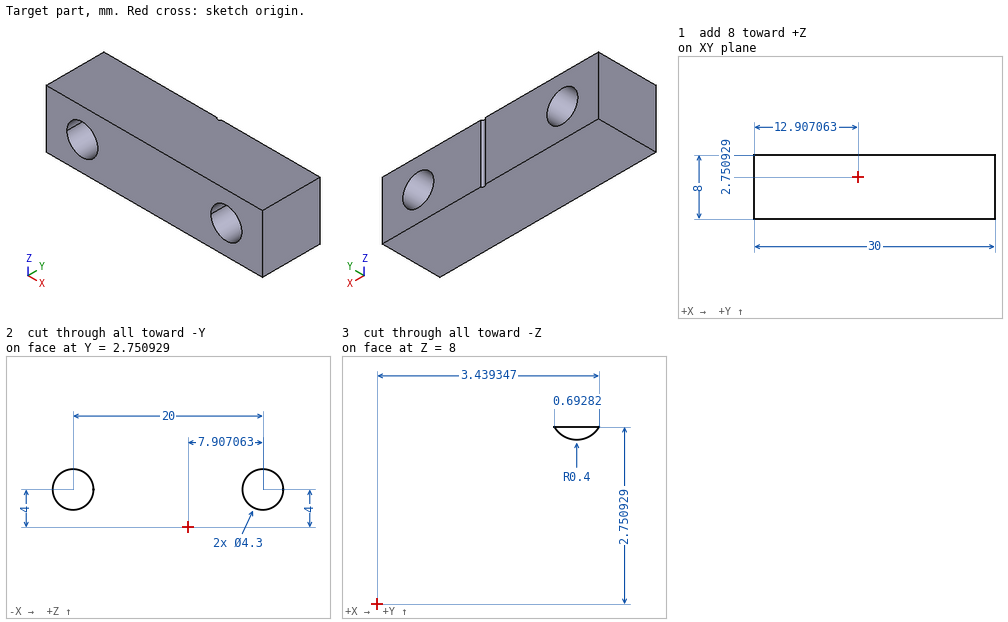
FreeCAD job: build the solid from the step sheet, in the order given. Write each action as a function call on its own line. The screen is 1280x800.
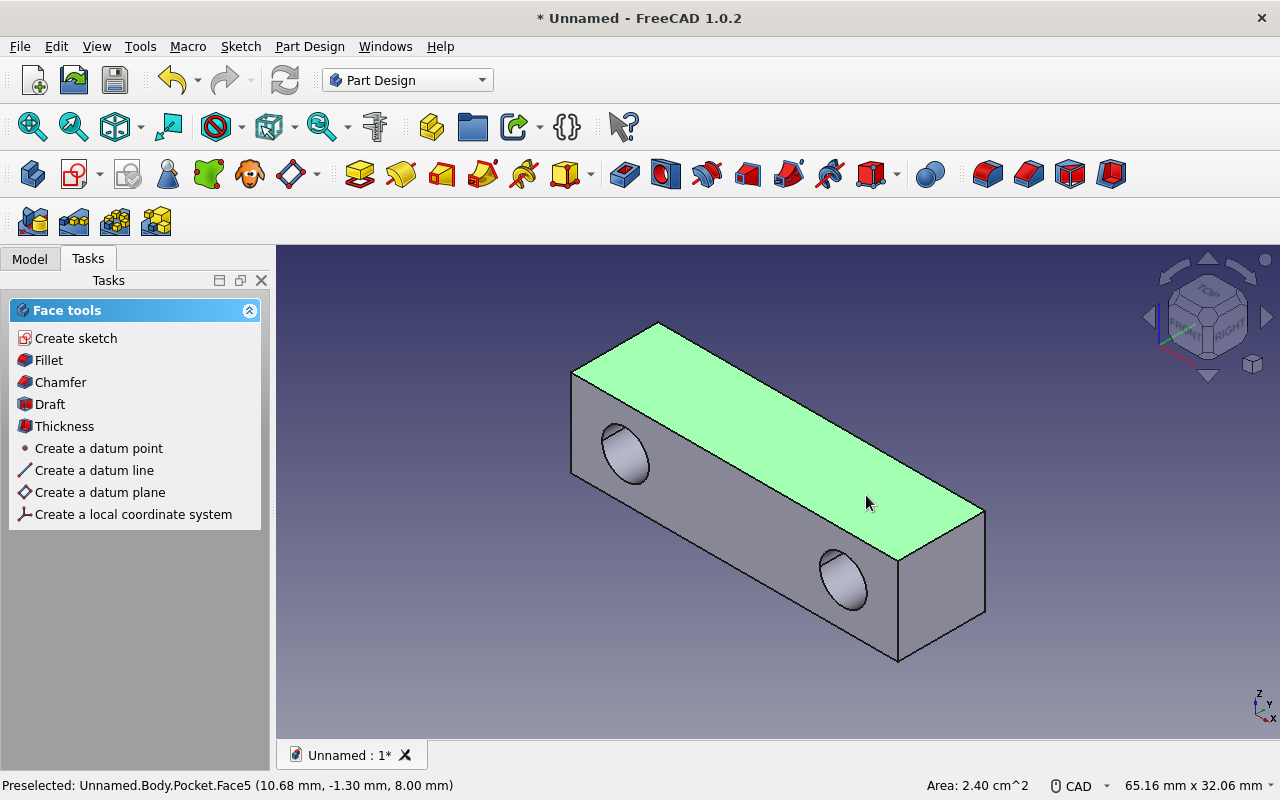
click(74, 174)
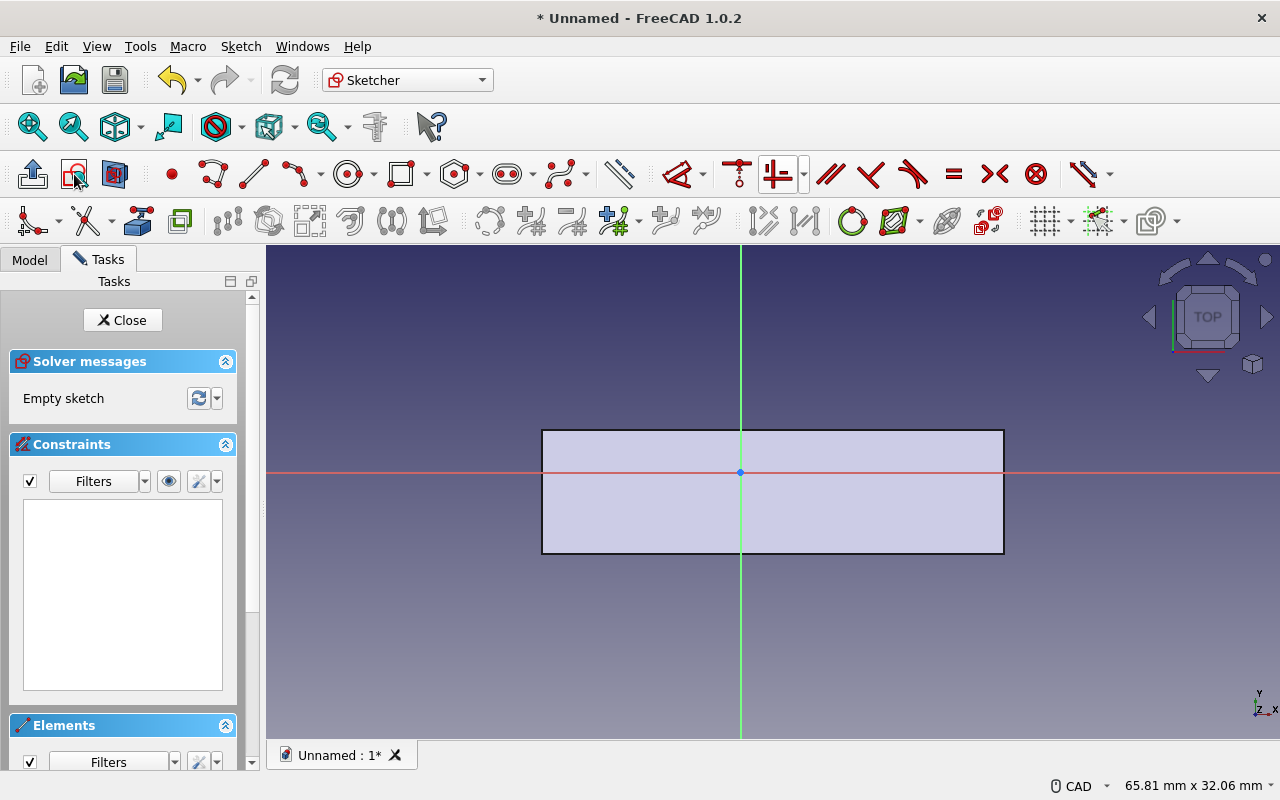
scroll(793, 429, up, 15)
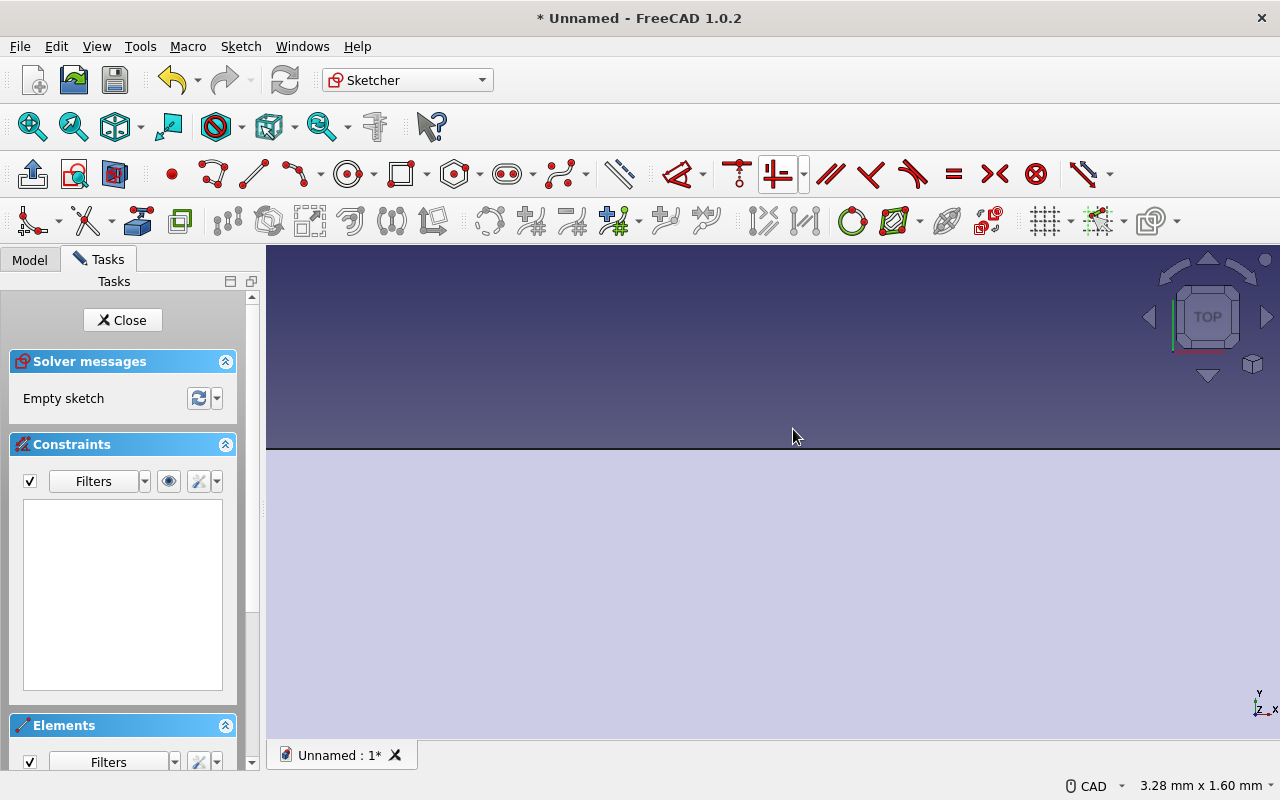
scroll(683, 474, up, 5)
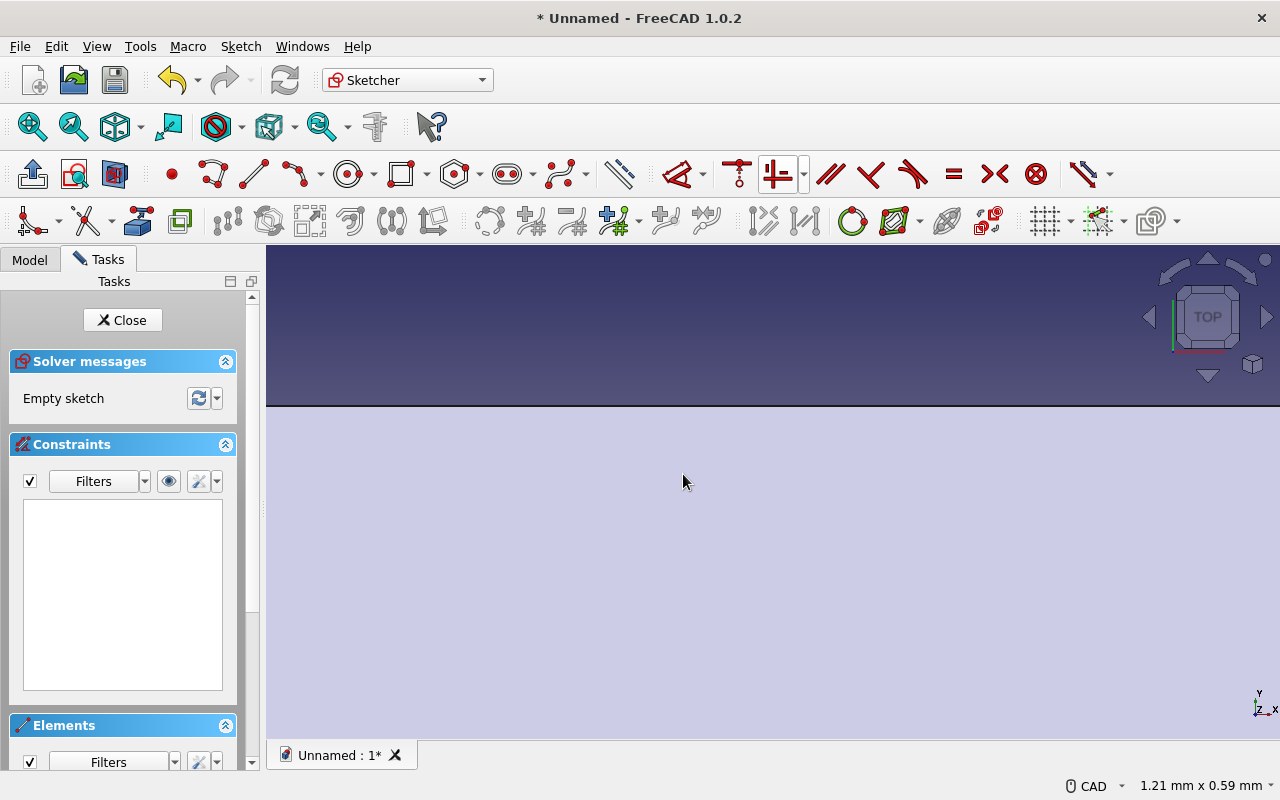
click(254, 174)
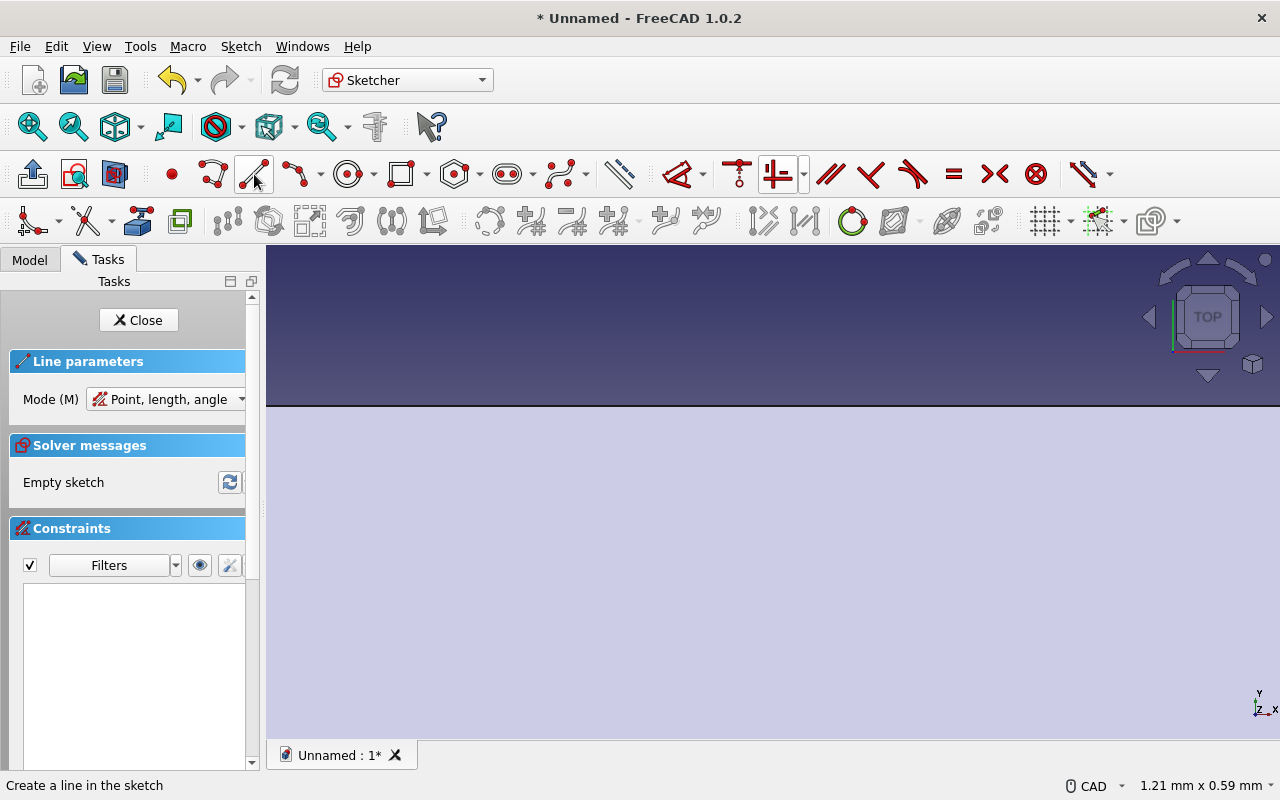
click(995, 406)
click(412, 406)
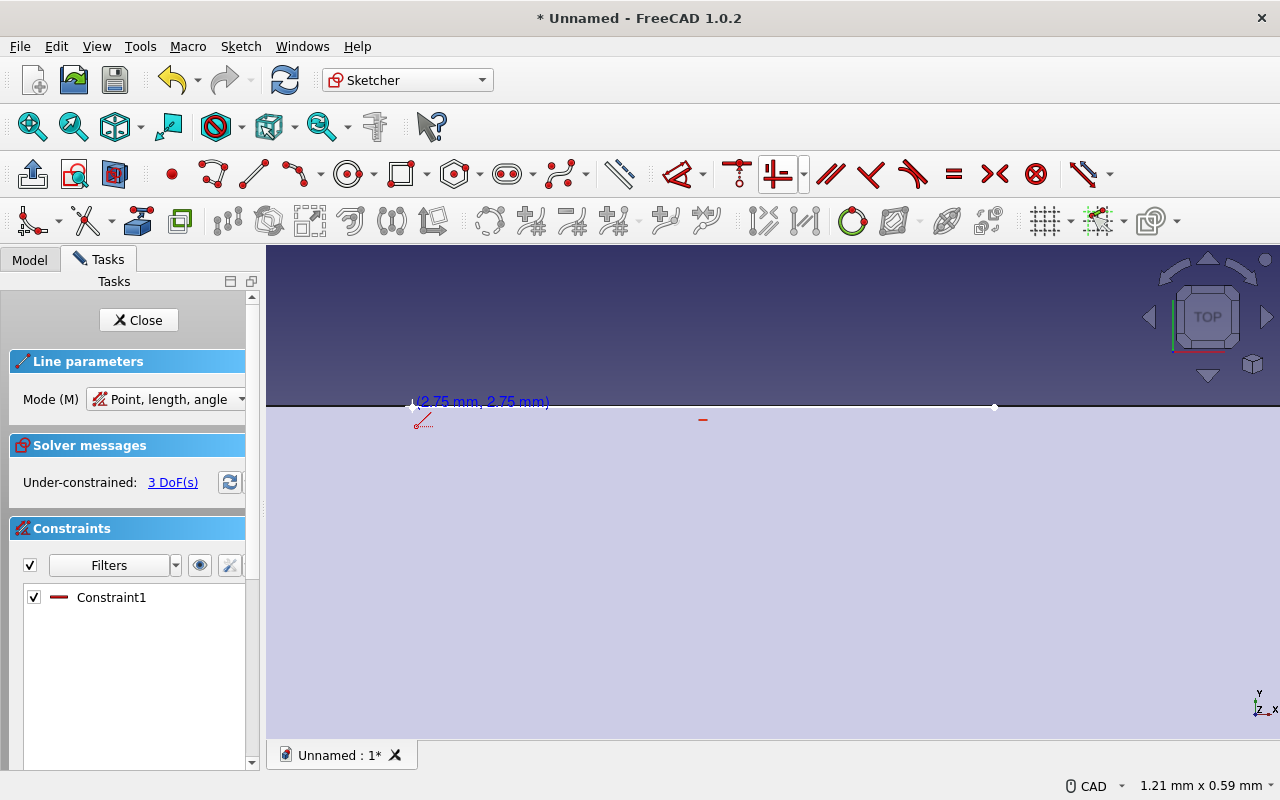
key(g)
key(3)
key(a)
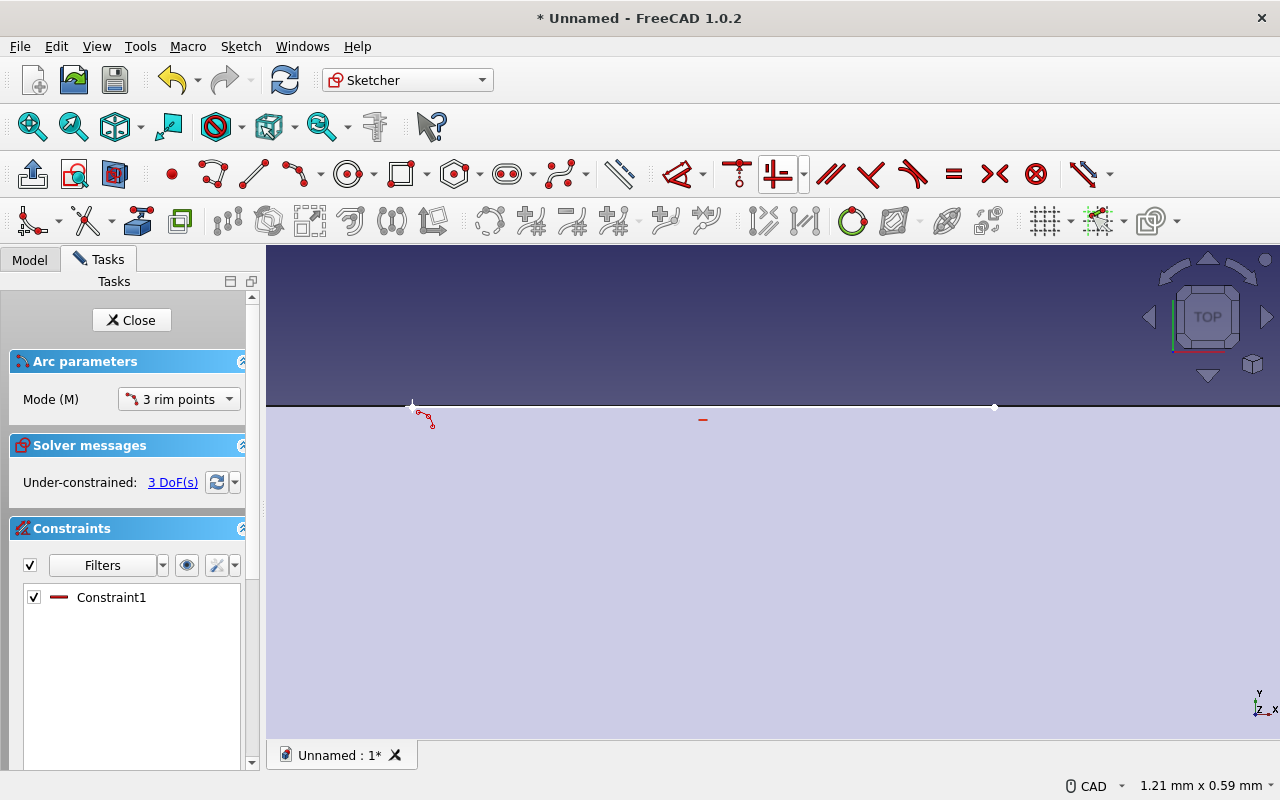
click(412, 407)
click(995, 407)
click(704, 575)
key(Escape)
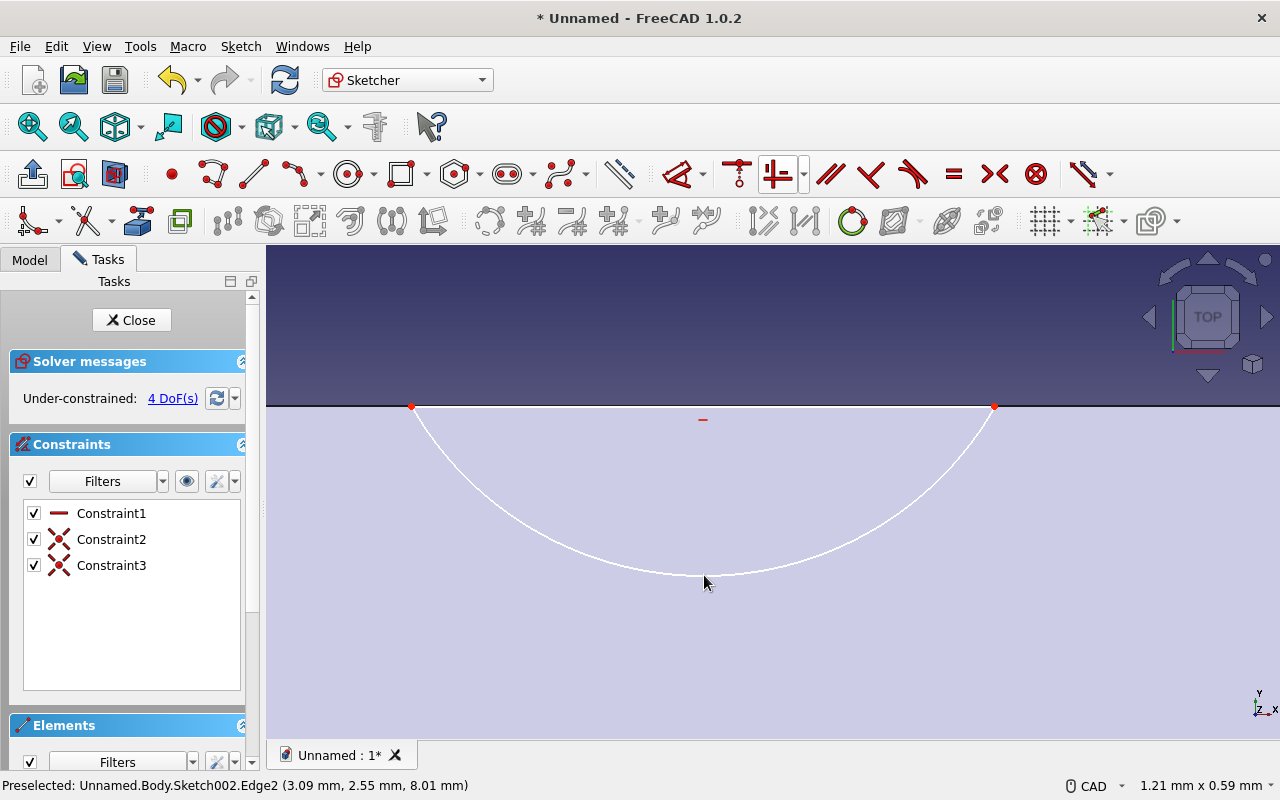
key(d)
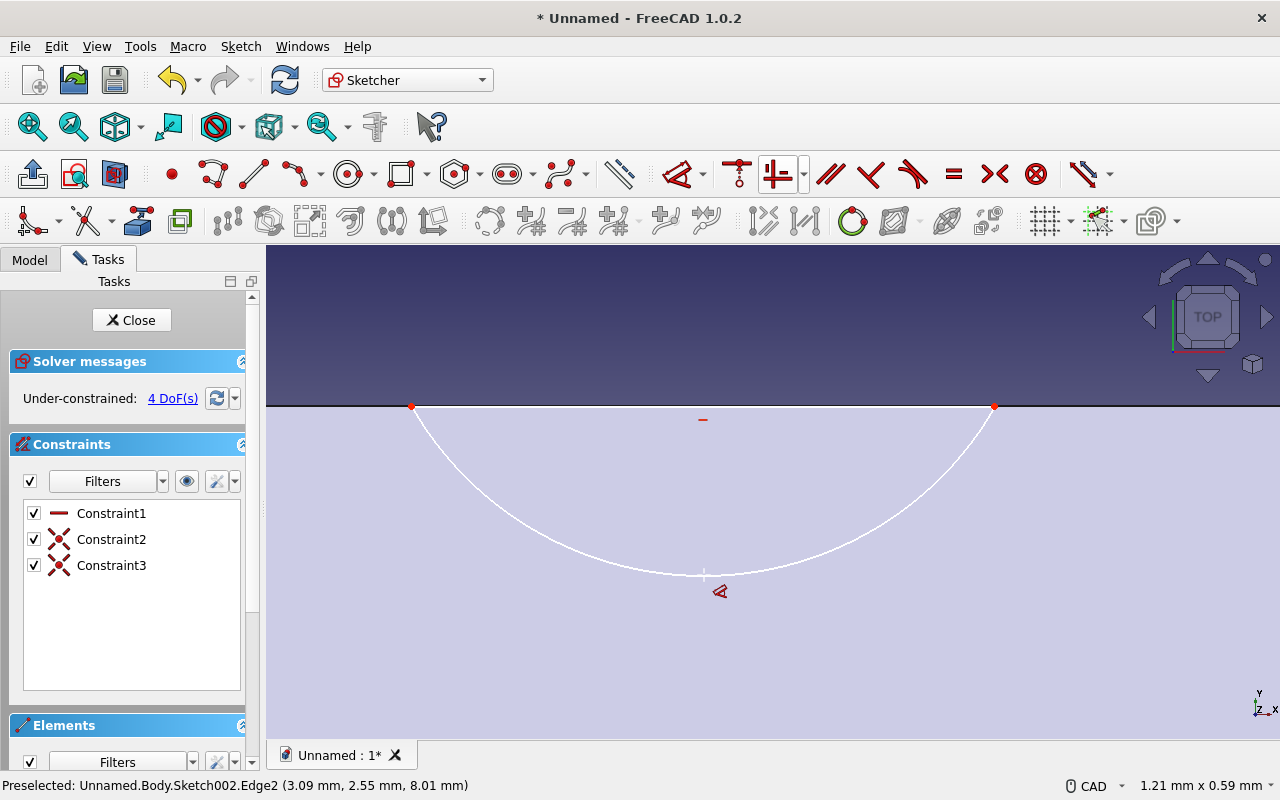
click(566, 547)
click(553, 576)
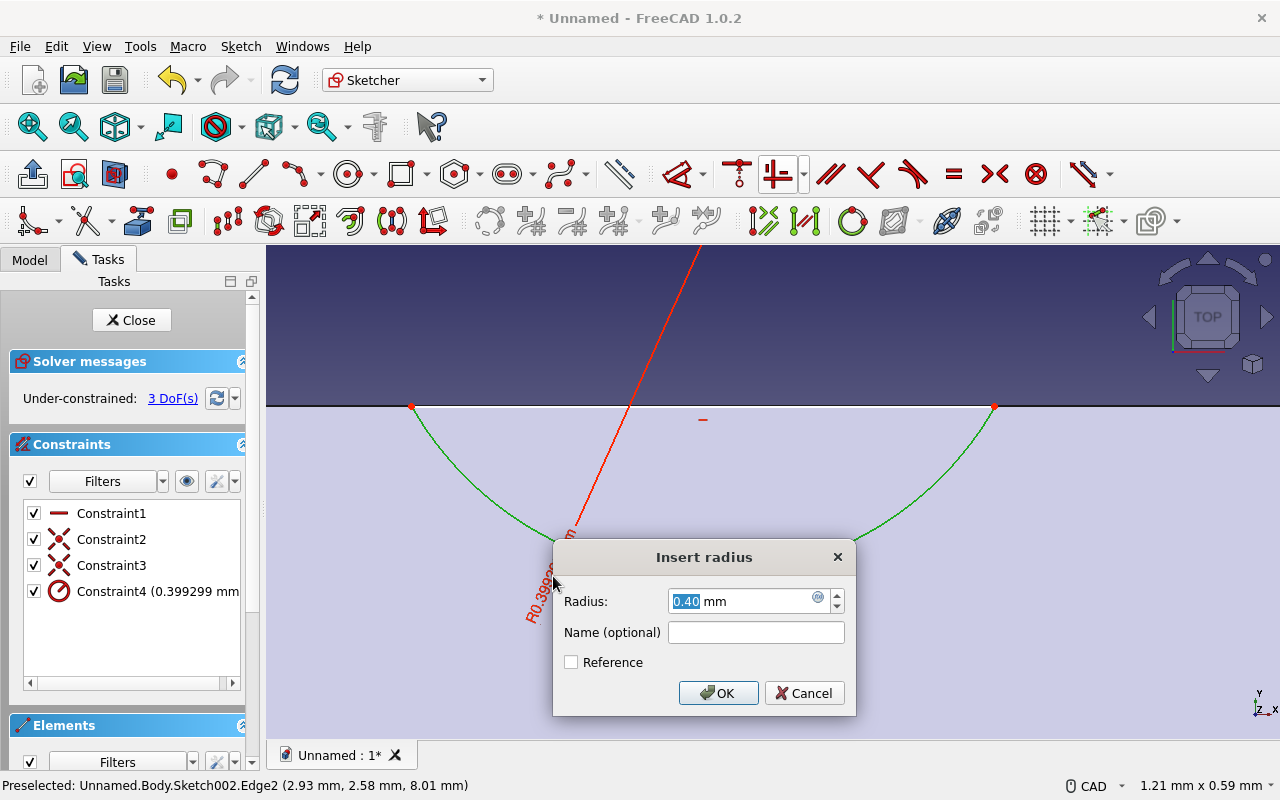
text(0.4)
key(Return)